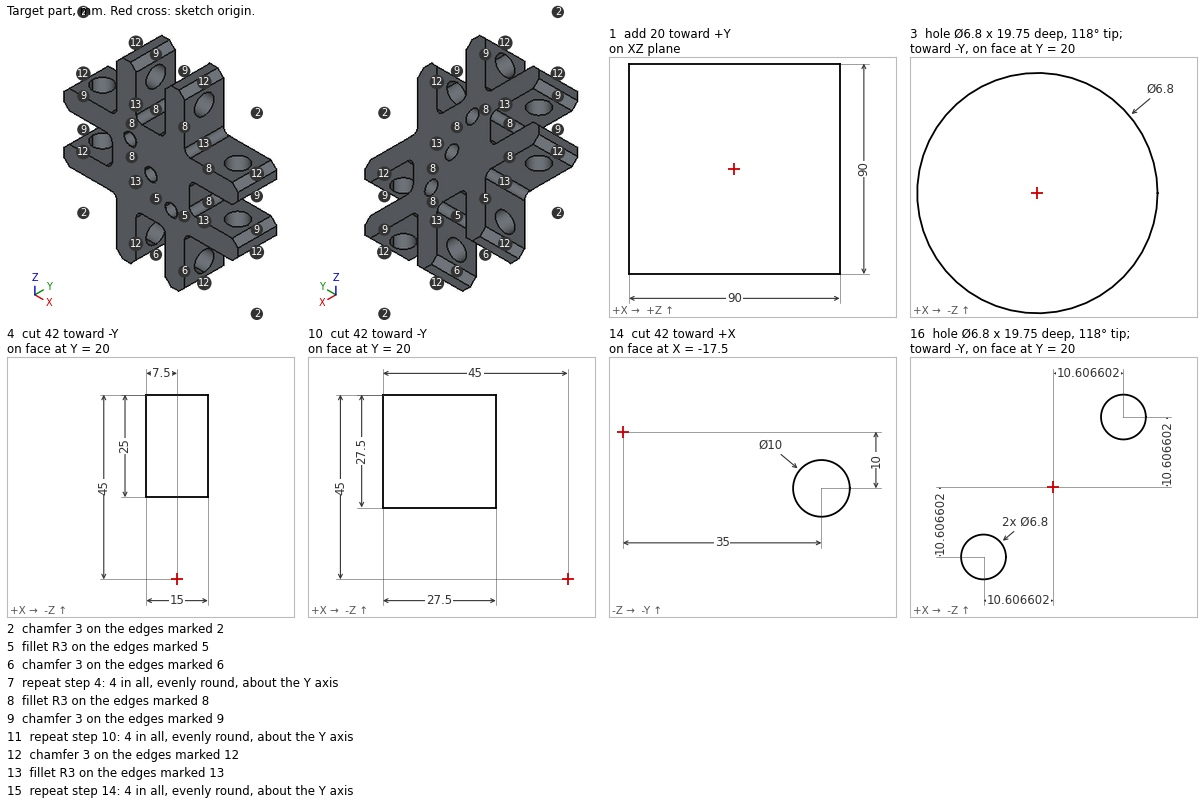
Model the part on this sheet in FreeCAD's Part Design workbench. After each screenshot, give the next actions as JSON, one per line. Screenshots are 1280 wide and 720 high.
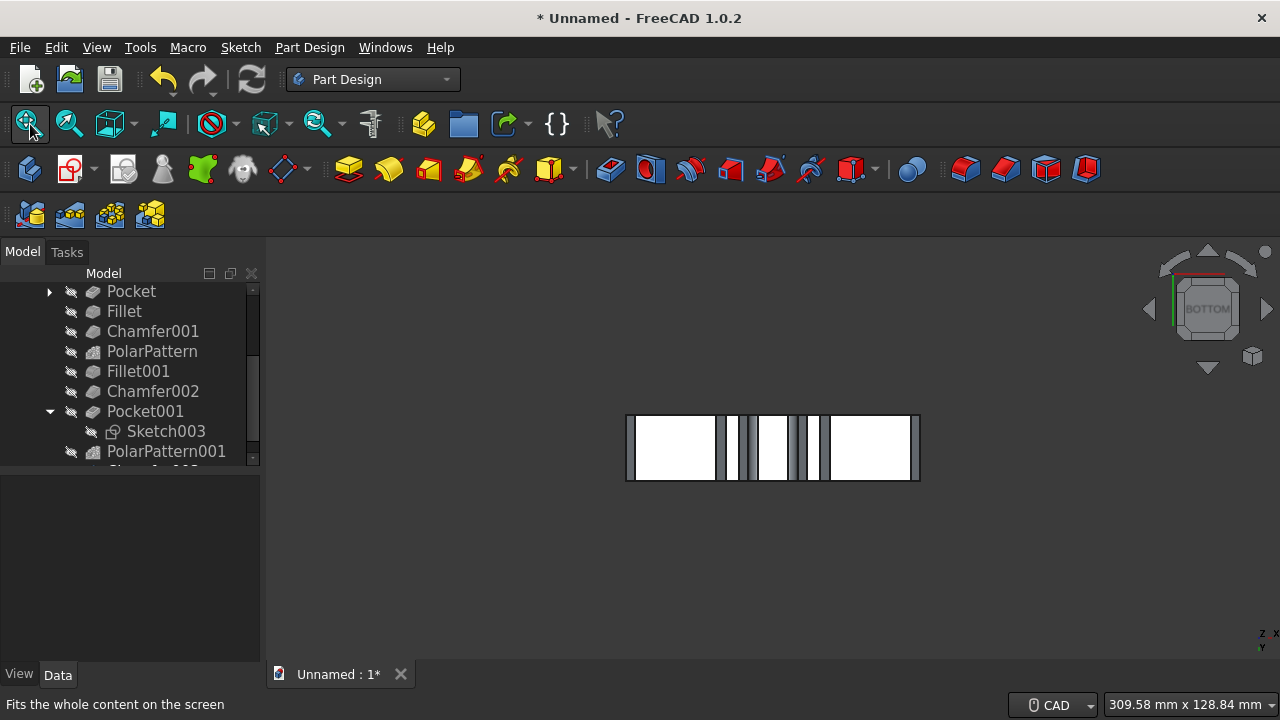
{"action": "key", "text": "0"}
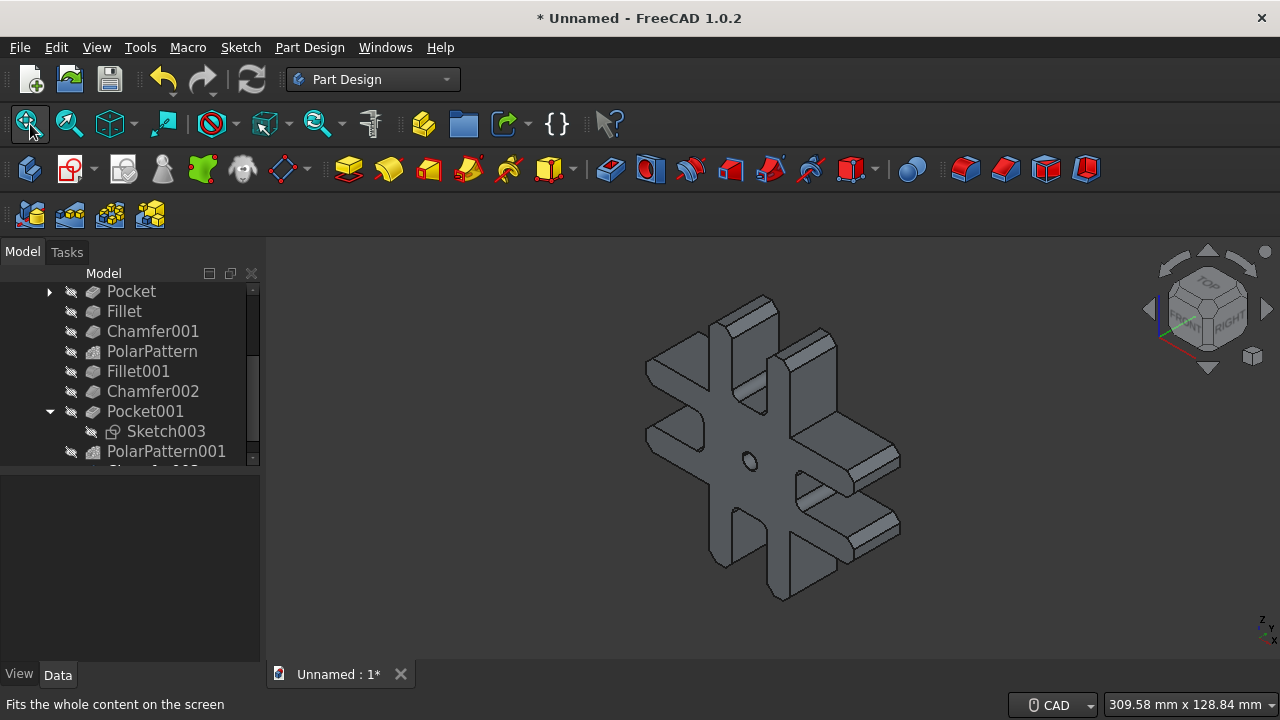
{"action": "key", "text": "2"}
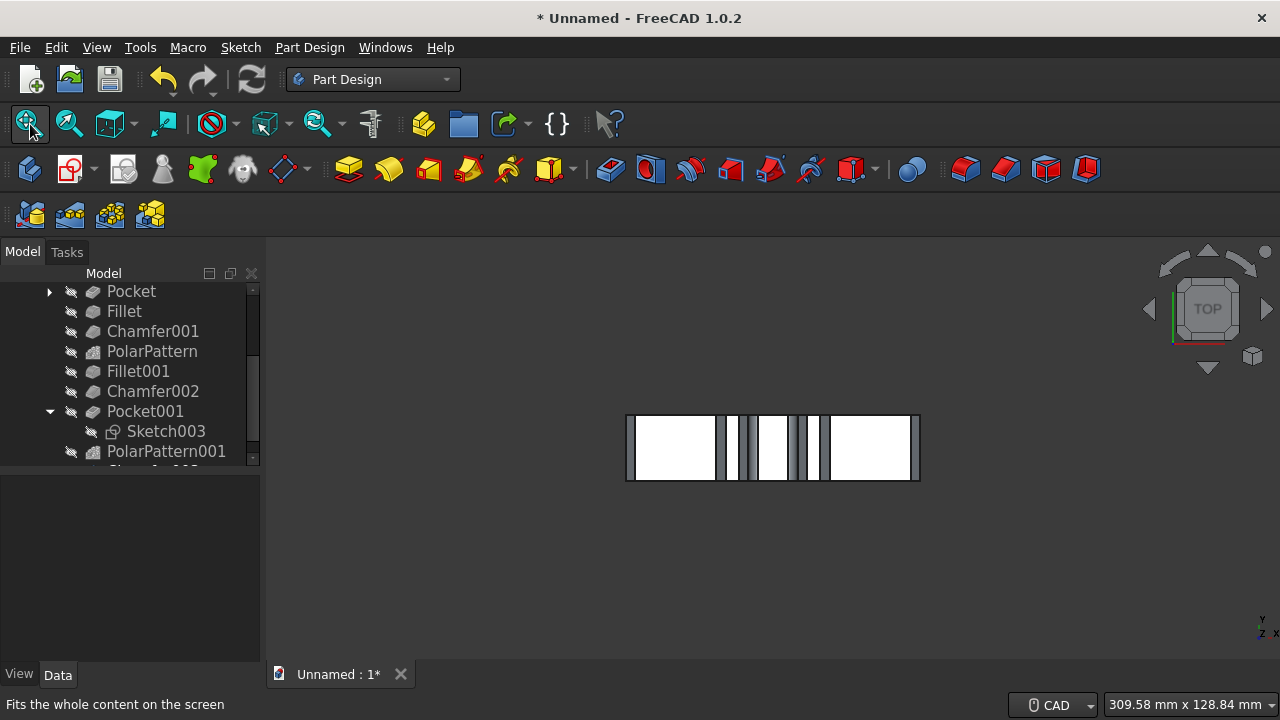
{"action": "left_click", "coordinate": [30, 124]}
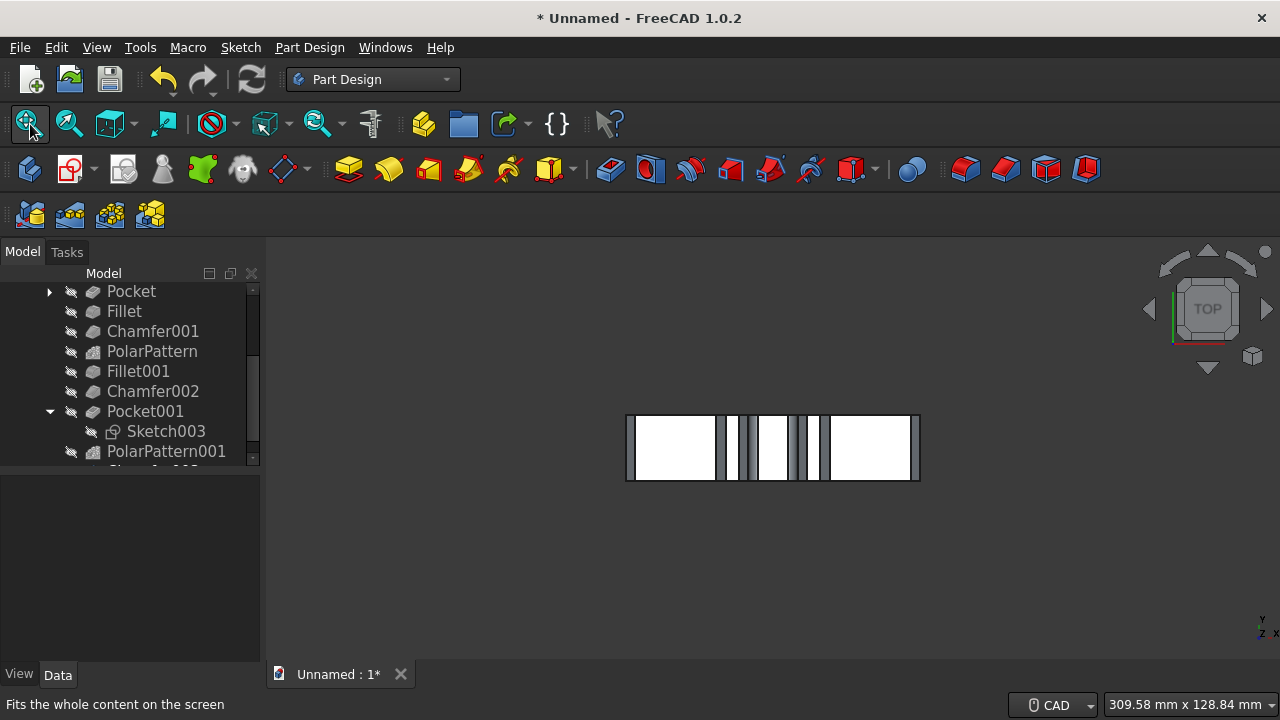
{"action": "key", "text": "1"}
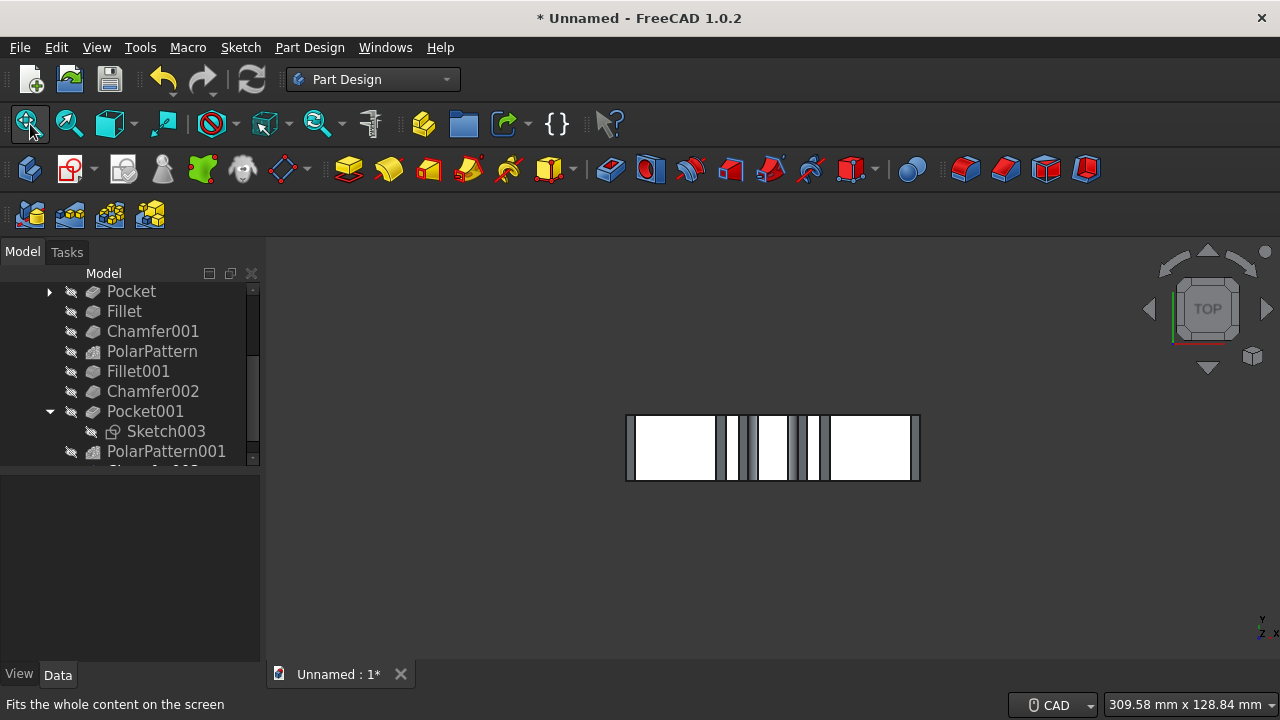
{"action": "key", "text": "3"}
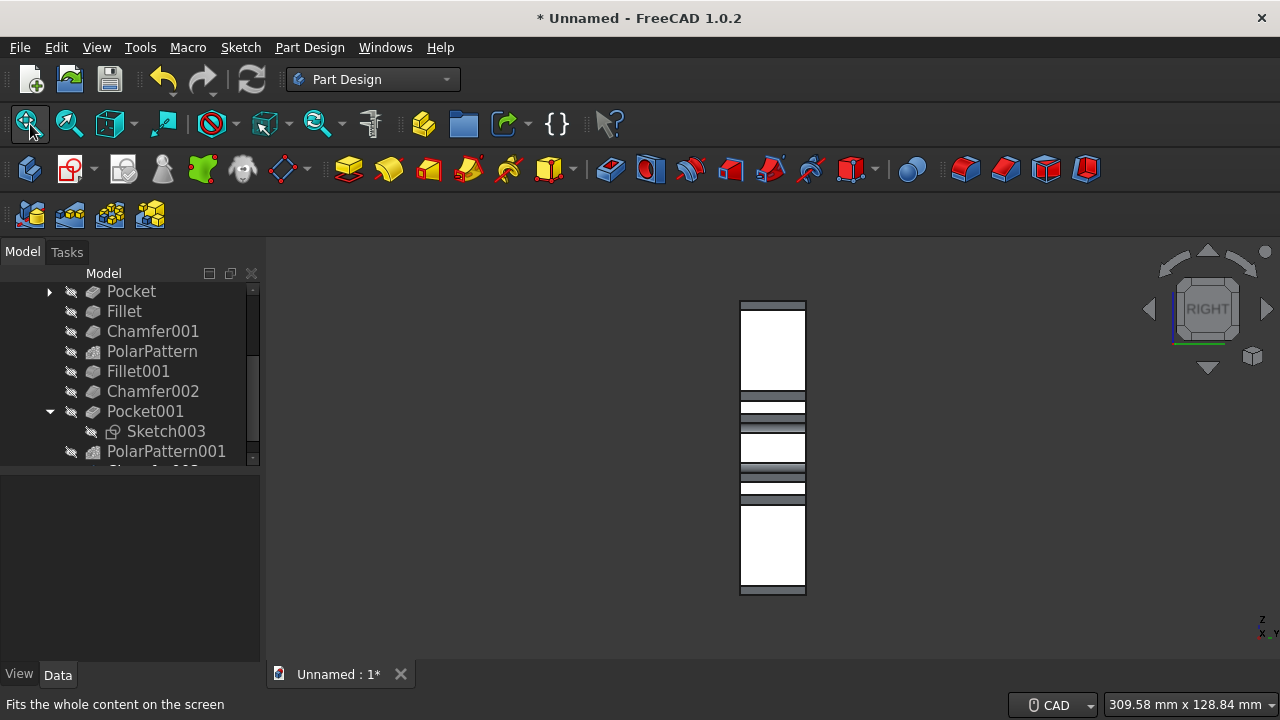
{"action": "key", "text": "5"}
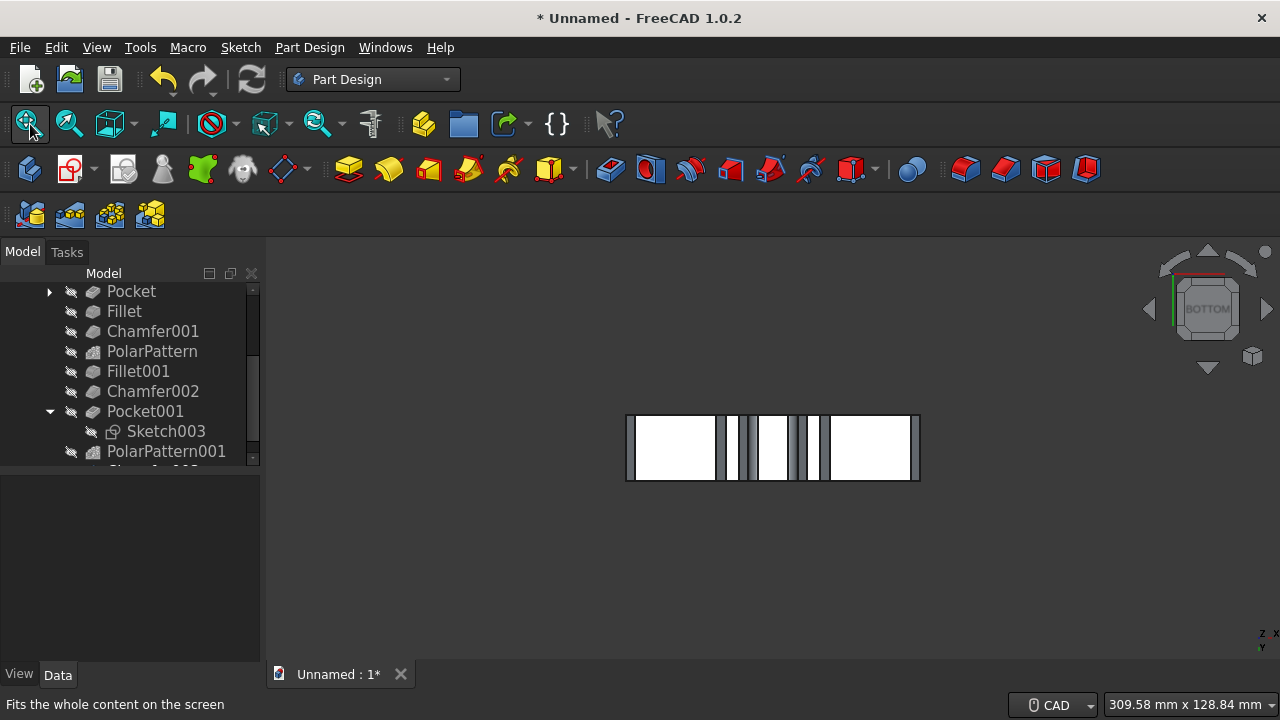
{"action": "left_click", "coordinate": [30, 124]}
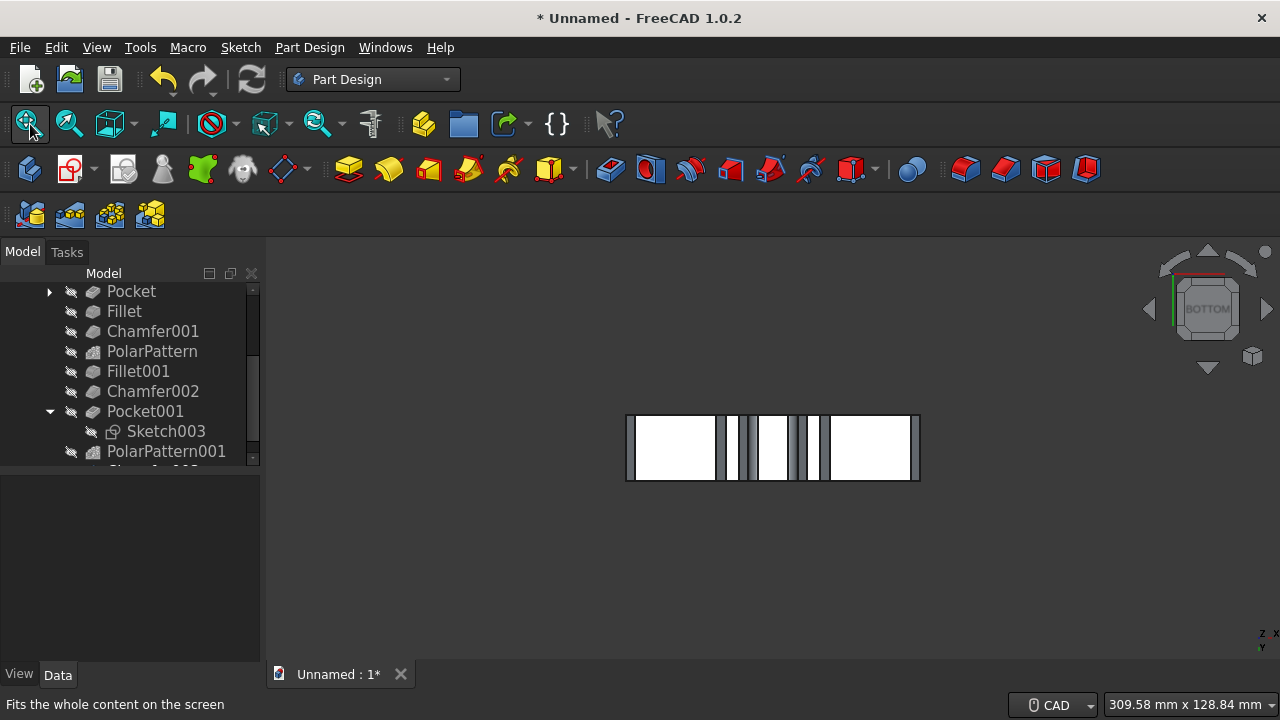
{"action": "key", "text": "4"}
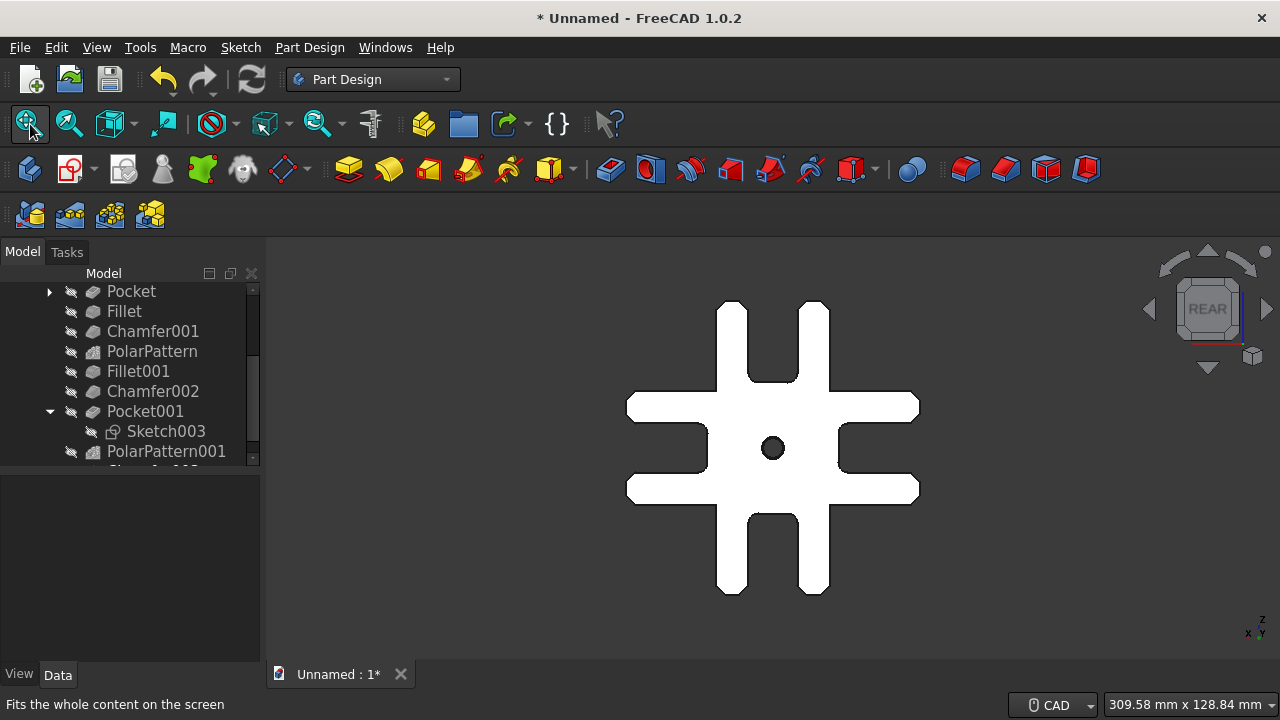
{"action": "key", "text": "6"}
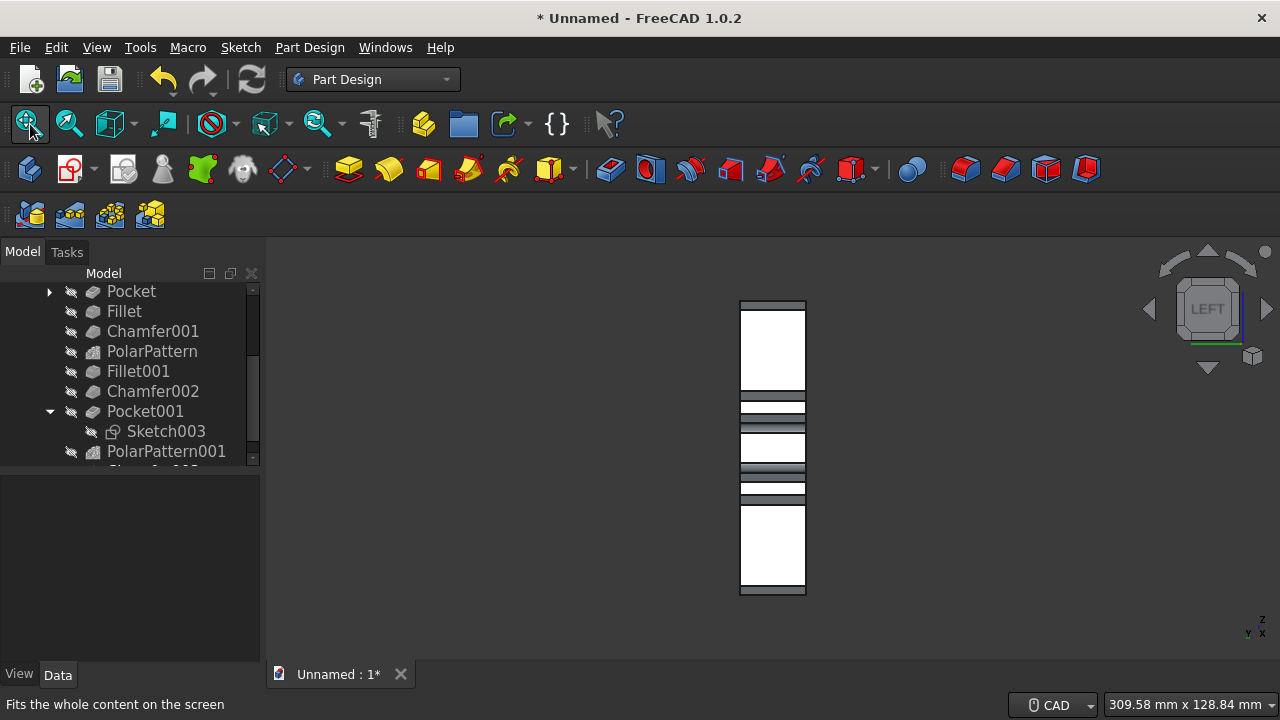
{"action": "key", "text": "v 3"}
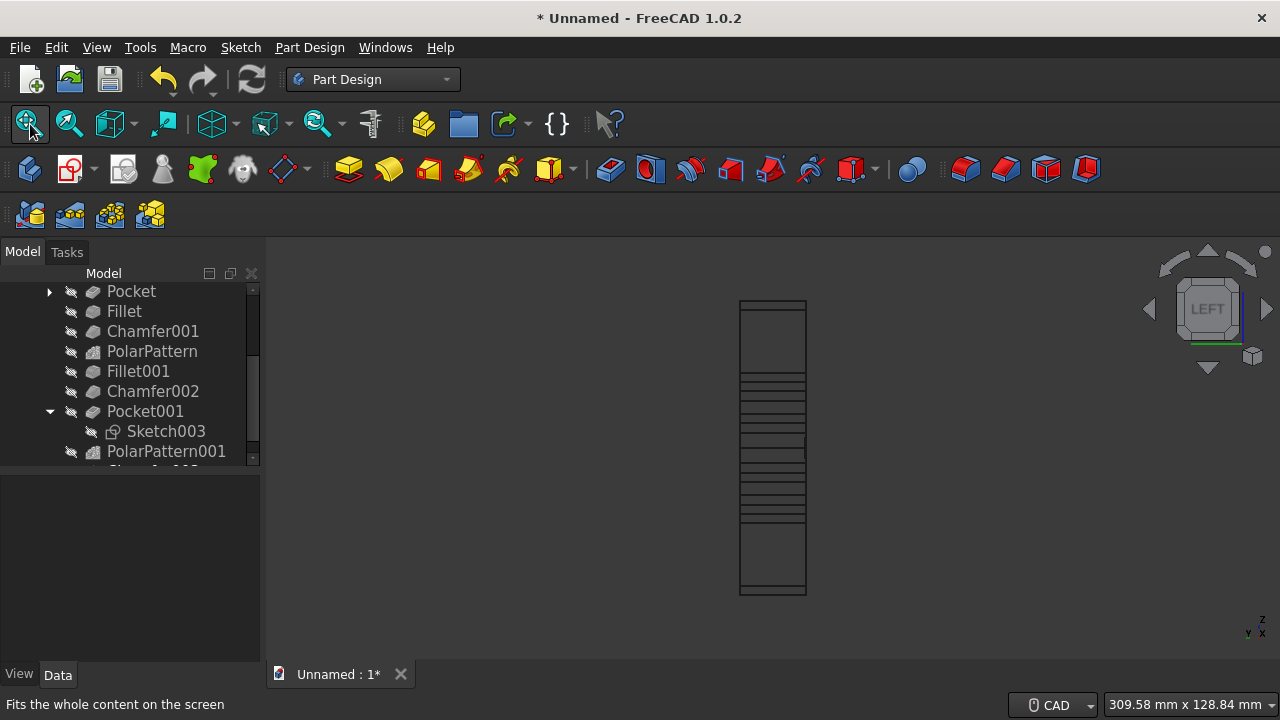
{"action": "key", "text": "0"}